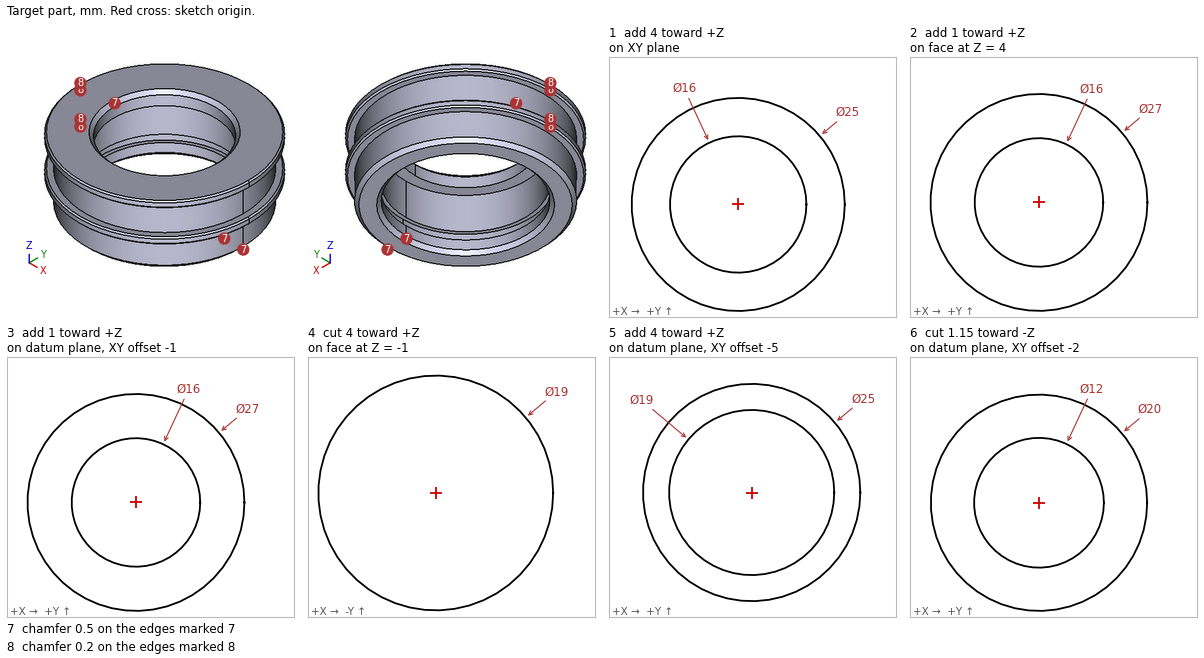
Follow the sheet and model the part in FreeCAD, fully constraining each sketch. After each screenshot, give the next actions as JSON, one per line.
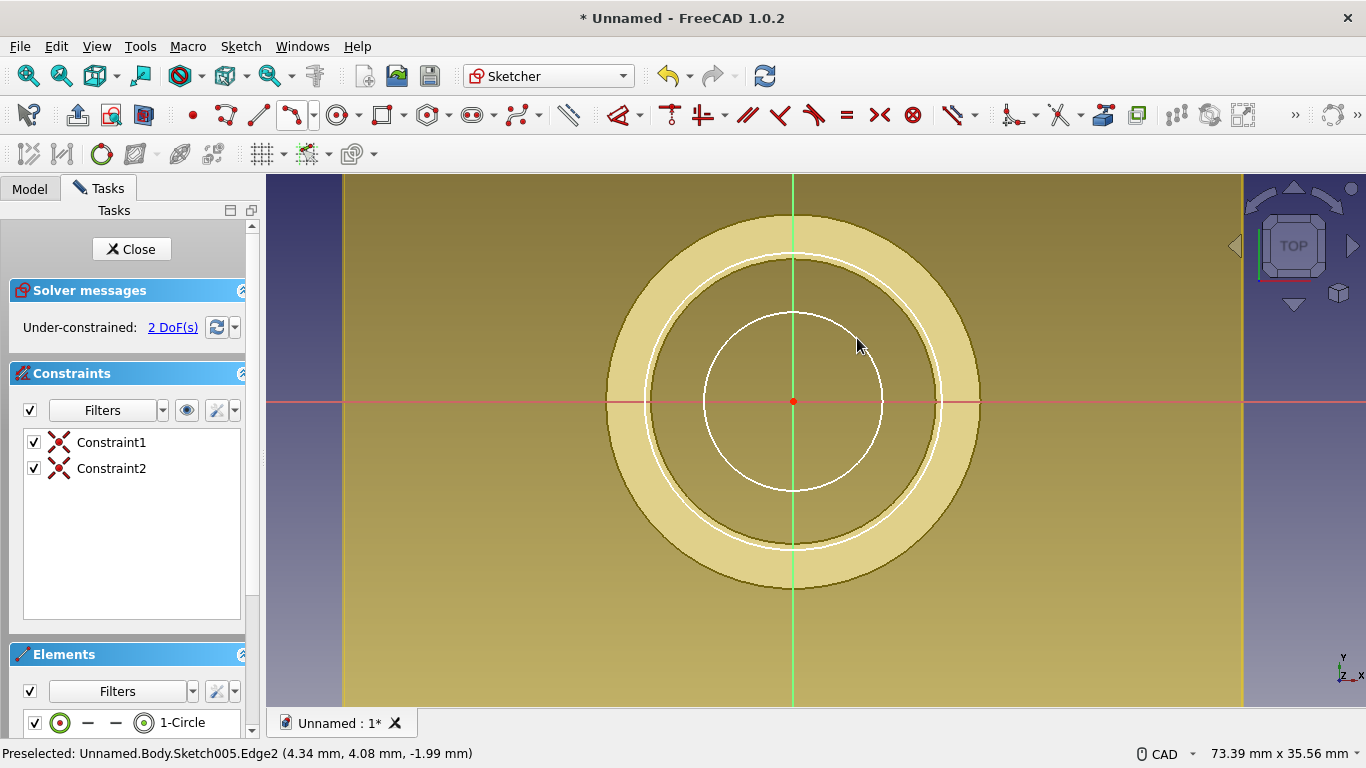
{"action": "left_click", "coordinate": [618, 116]}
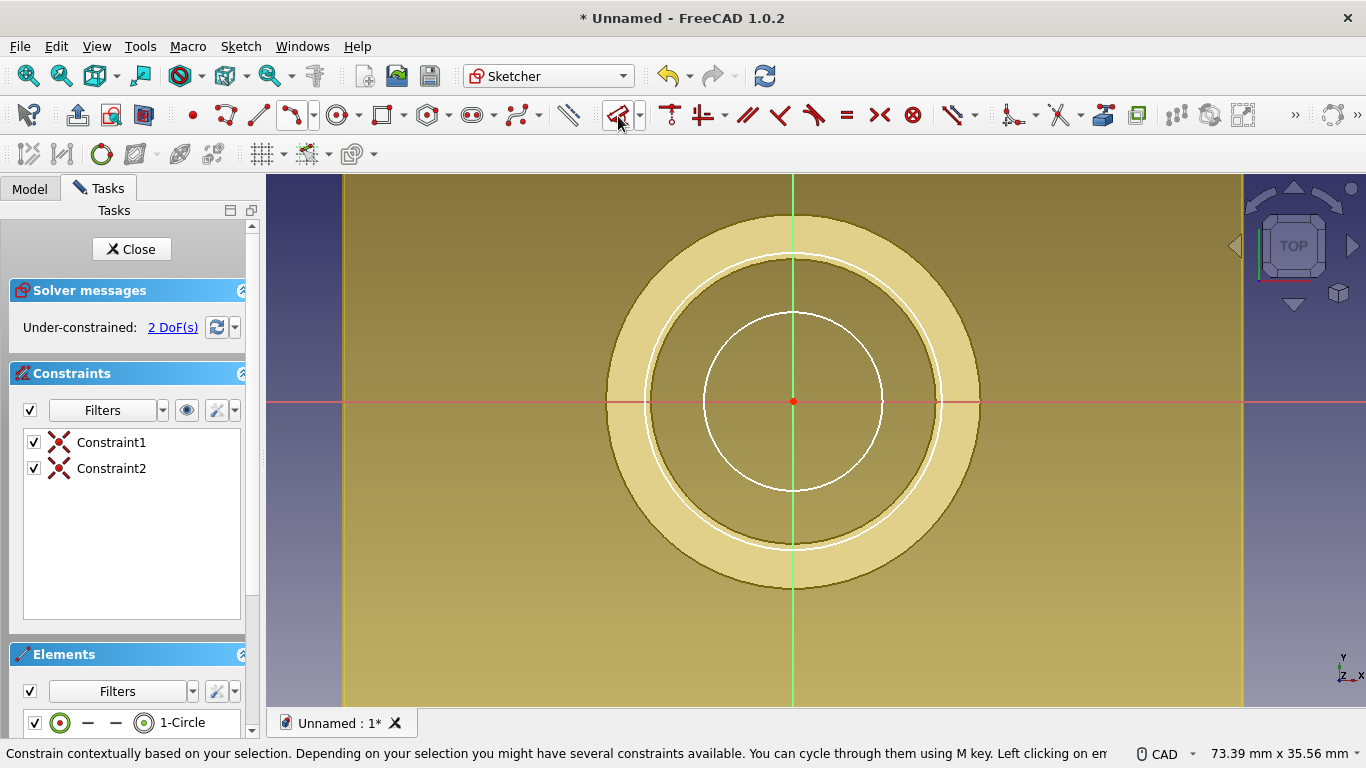
{"action": "left_click", "coordinate": [898, 296]}
{"action": "left_click", "coordinate": [921, 273]}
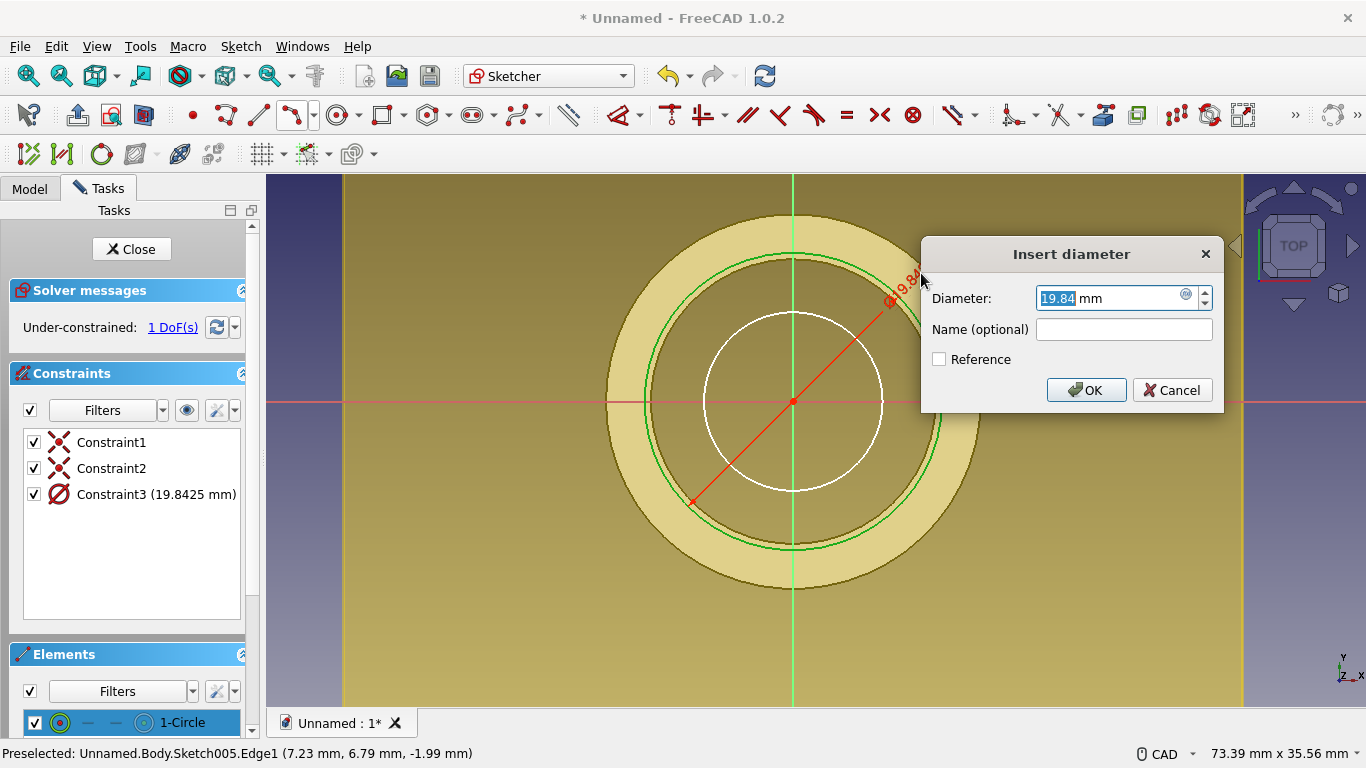
{"action": "type", "text": "20"}
{"action": "key", "text": "Return"}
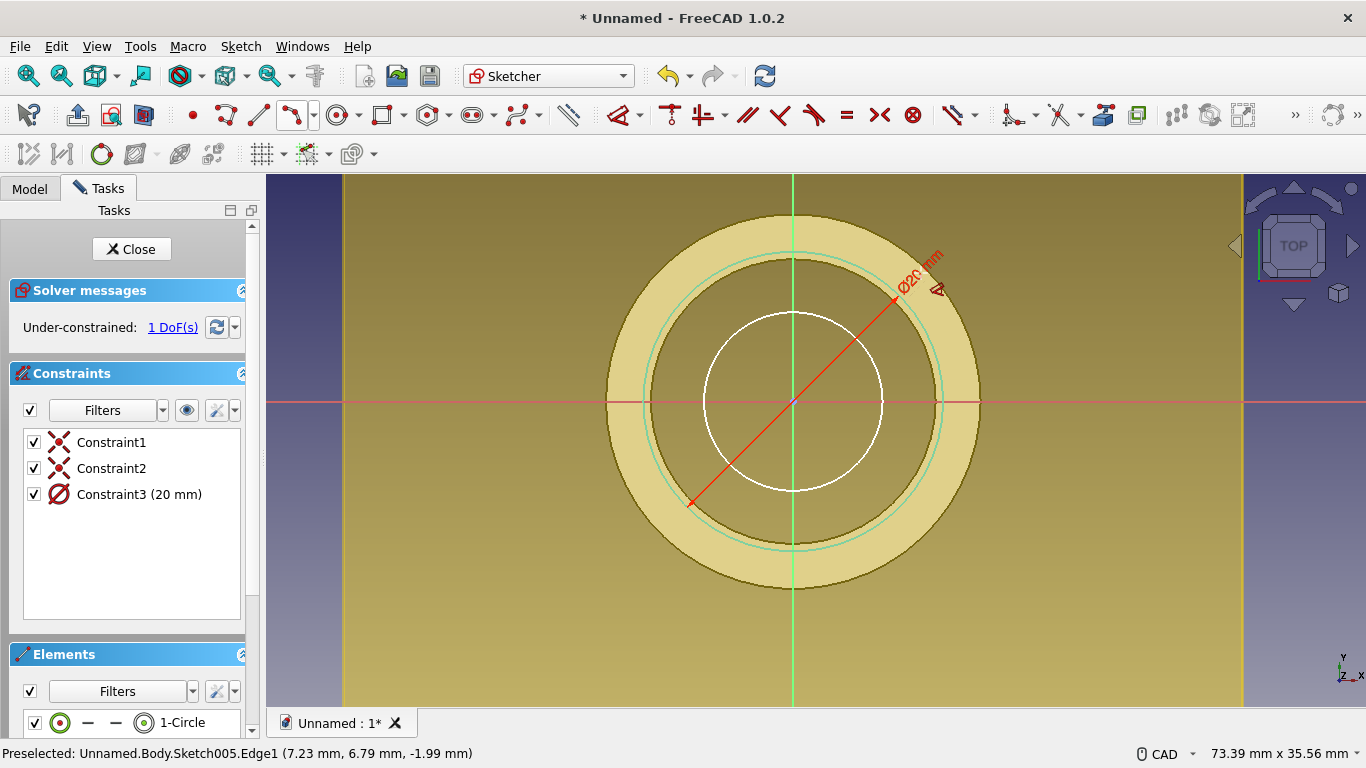
{"action": "left_click", "coordinate": [856, 338]}
{"action": "left_click", "coordinate": [878, 315]}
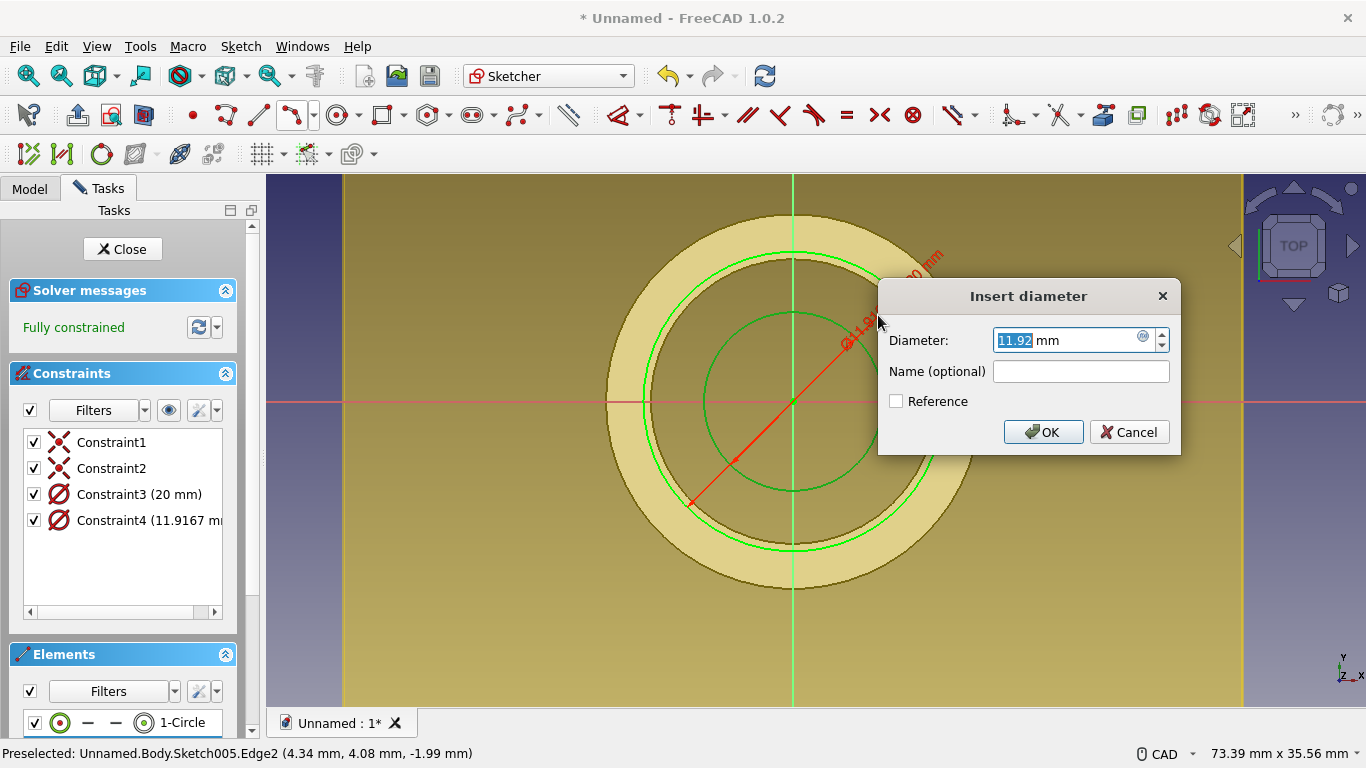
{"action": "type", "text": "12"}
{"action": "key", "text": "Return"}
{"action": "key", "text": "Escape"}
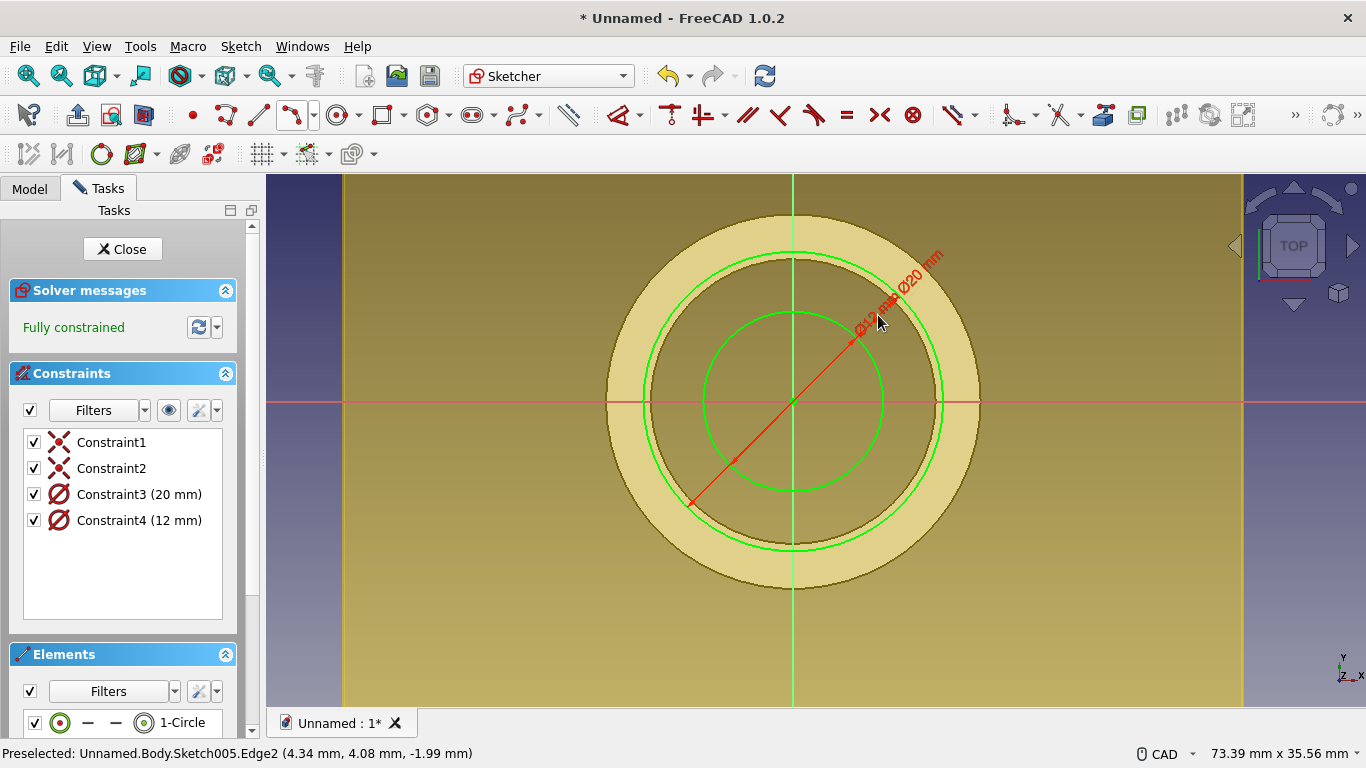
{"action": "left_click", "coordinate": [123, 249]}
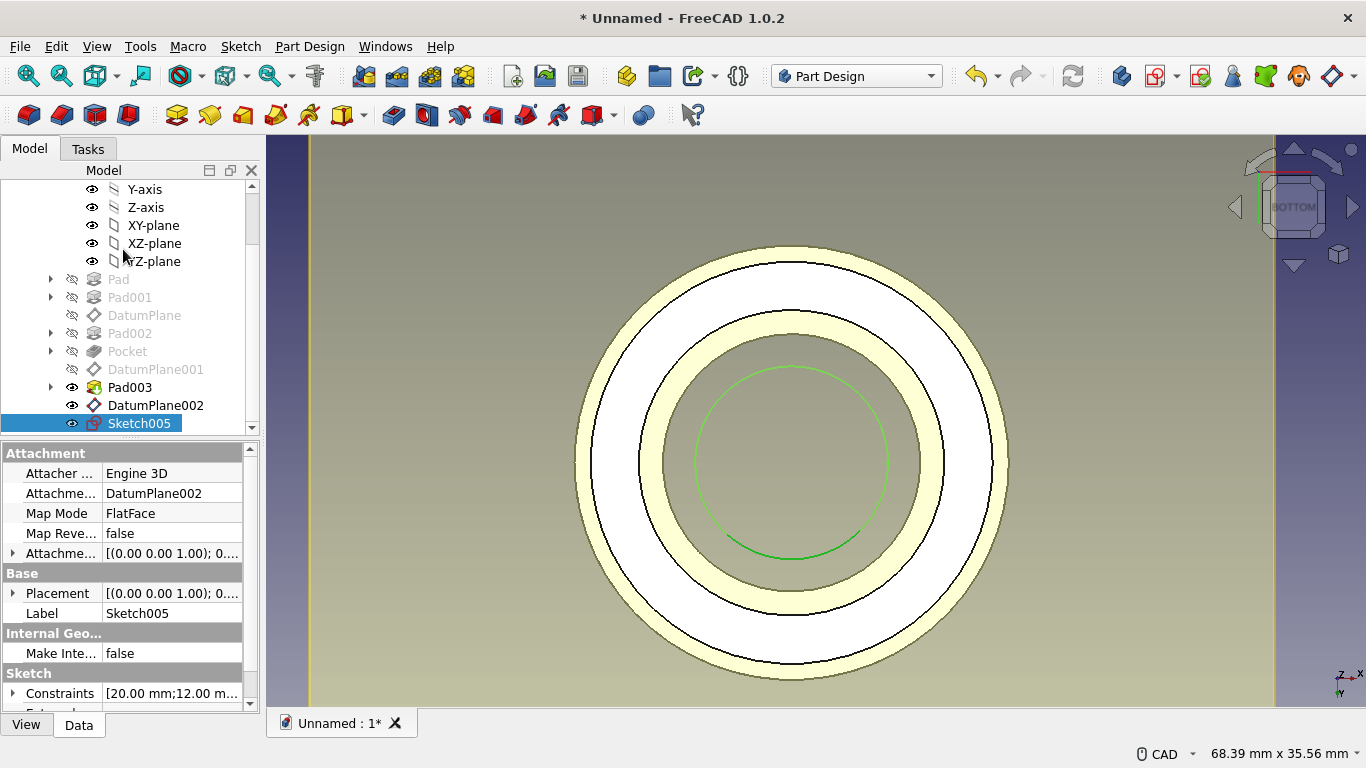
{"action": "left_click", "coordinate": [394, 116]}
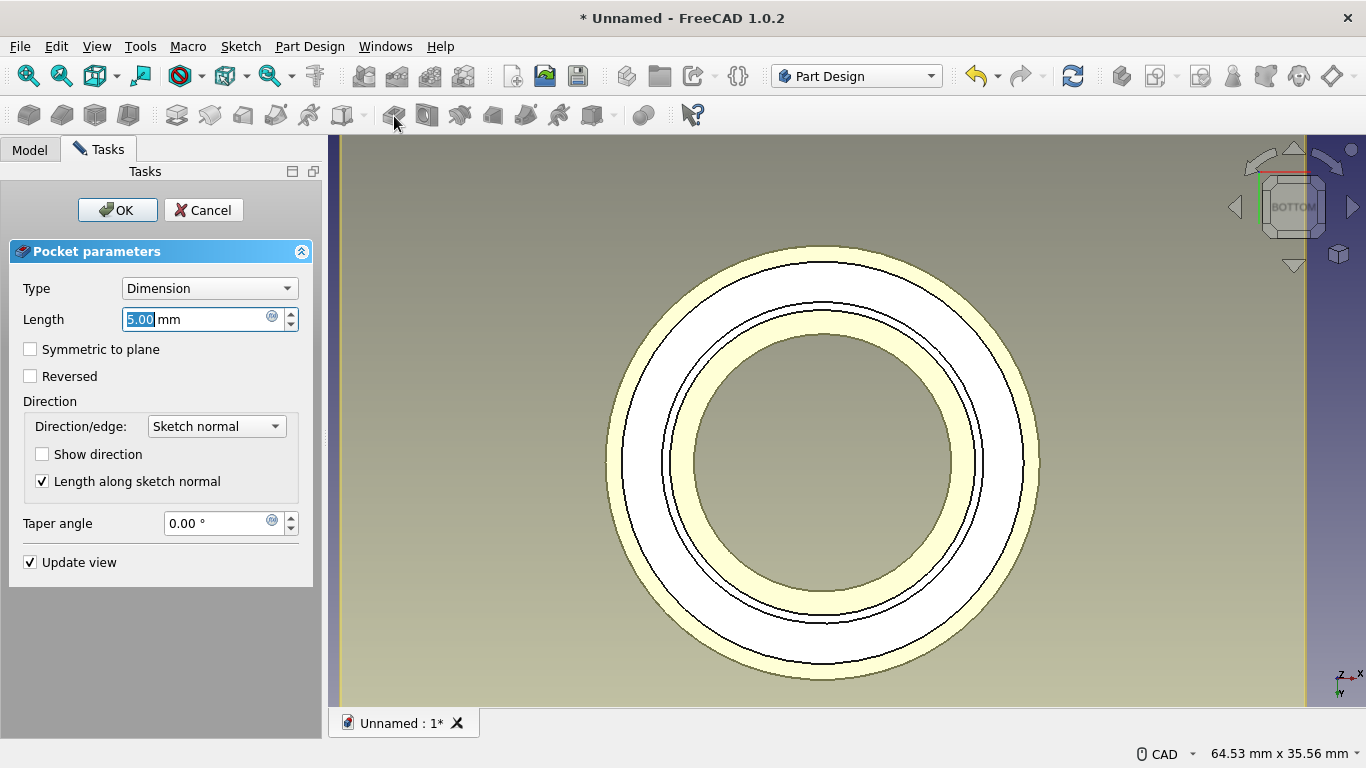
{"action": "type", "text": "1.15"}
{"action": "key", "text": "Tab"}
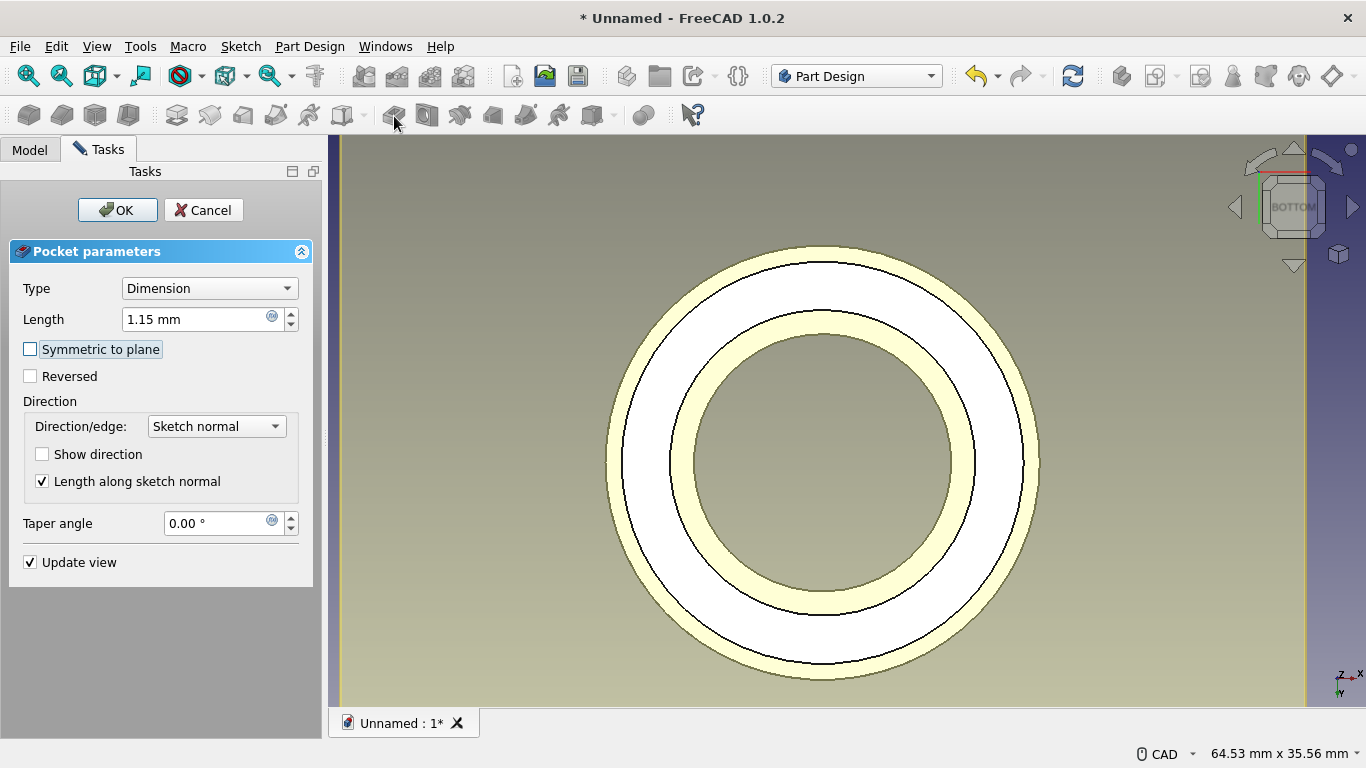
{"action": "left_click", "coordinate": [118, 210]}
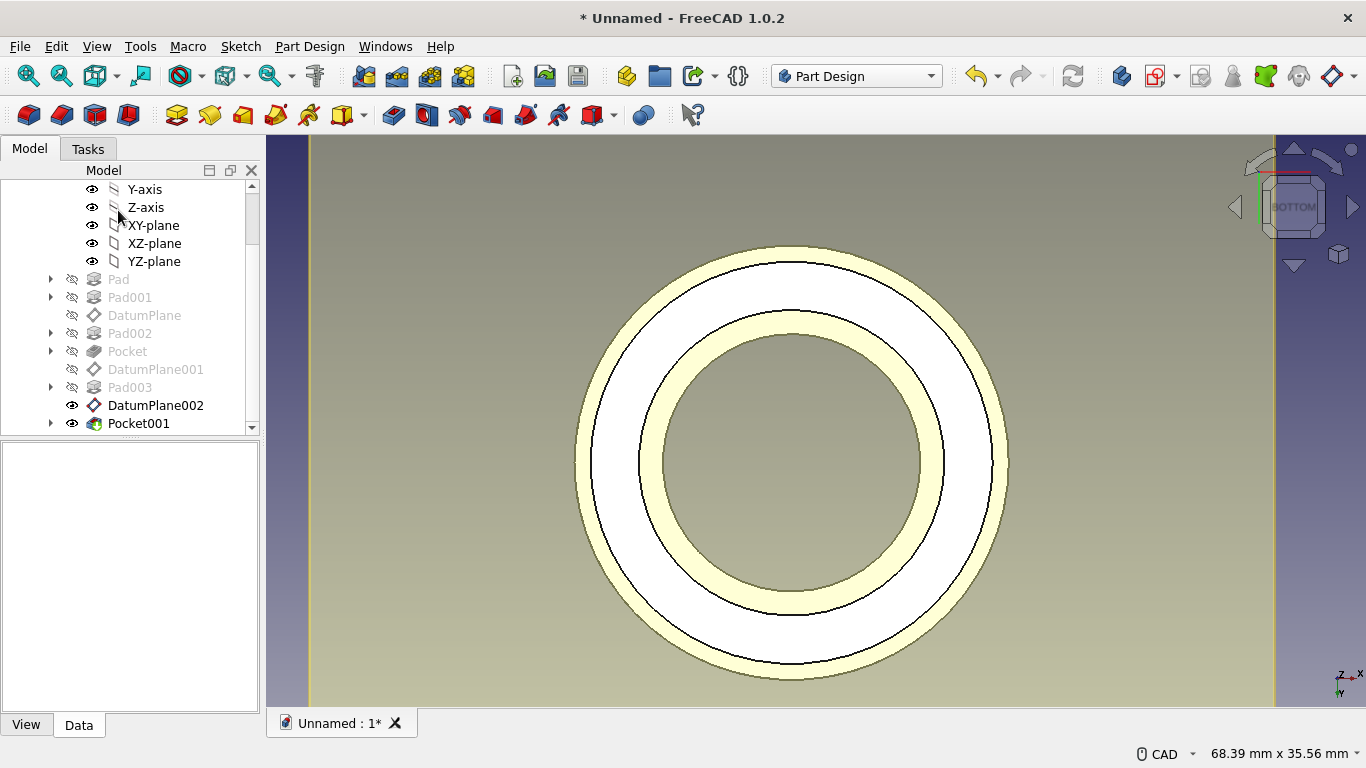
{"action": "left_click", "coordinate": [117, 405]}
{"action": "key", "text": "space"}